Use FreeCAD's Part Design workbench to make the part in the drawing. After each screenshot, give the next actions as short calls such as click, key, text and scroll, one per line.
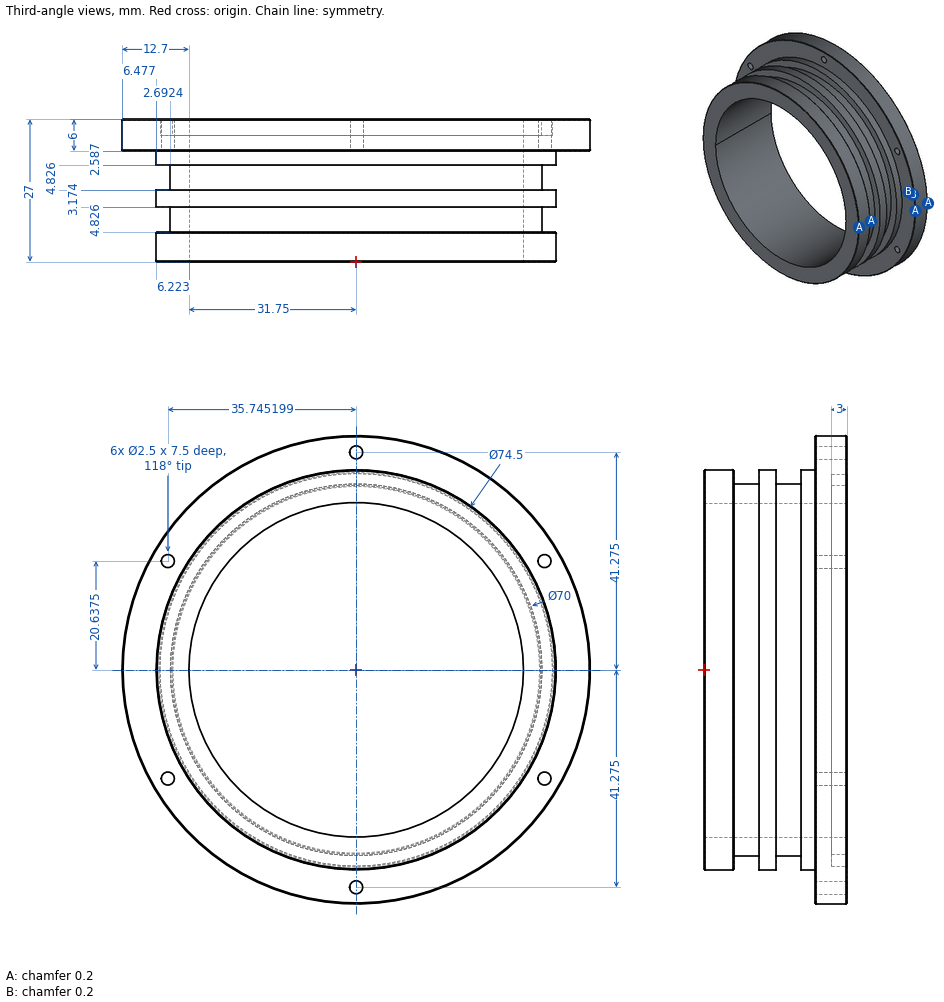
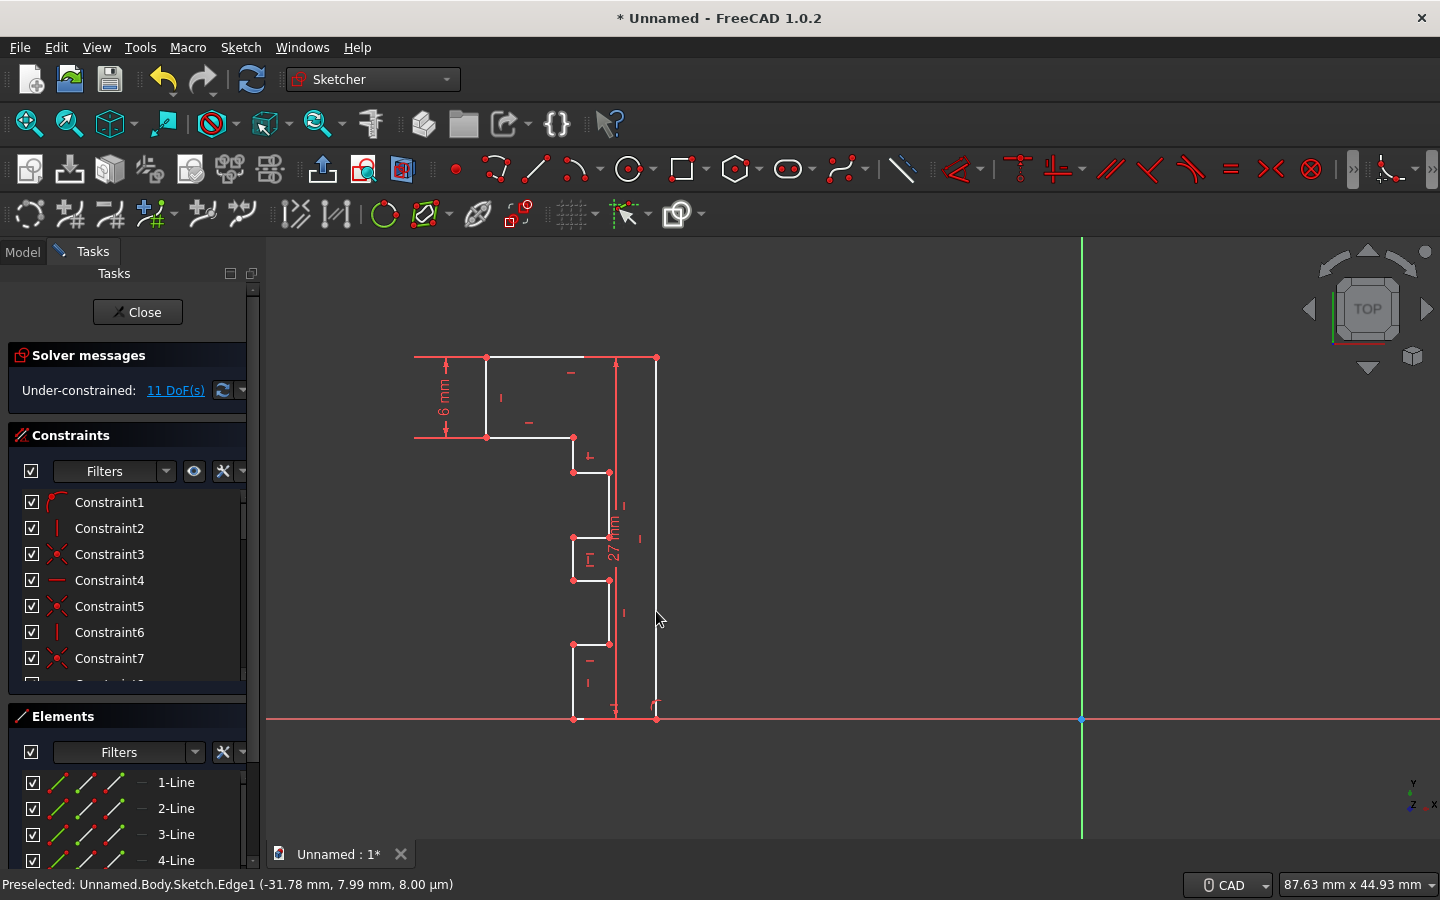
click(605, 357)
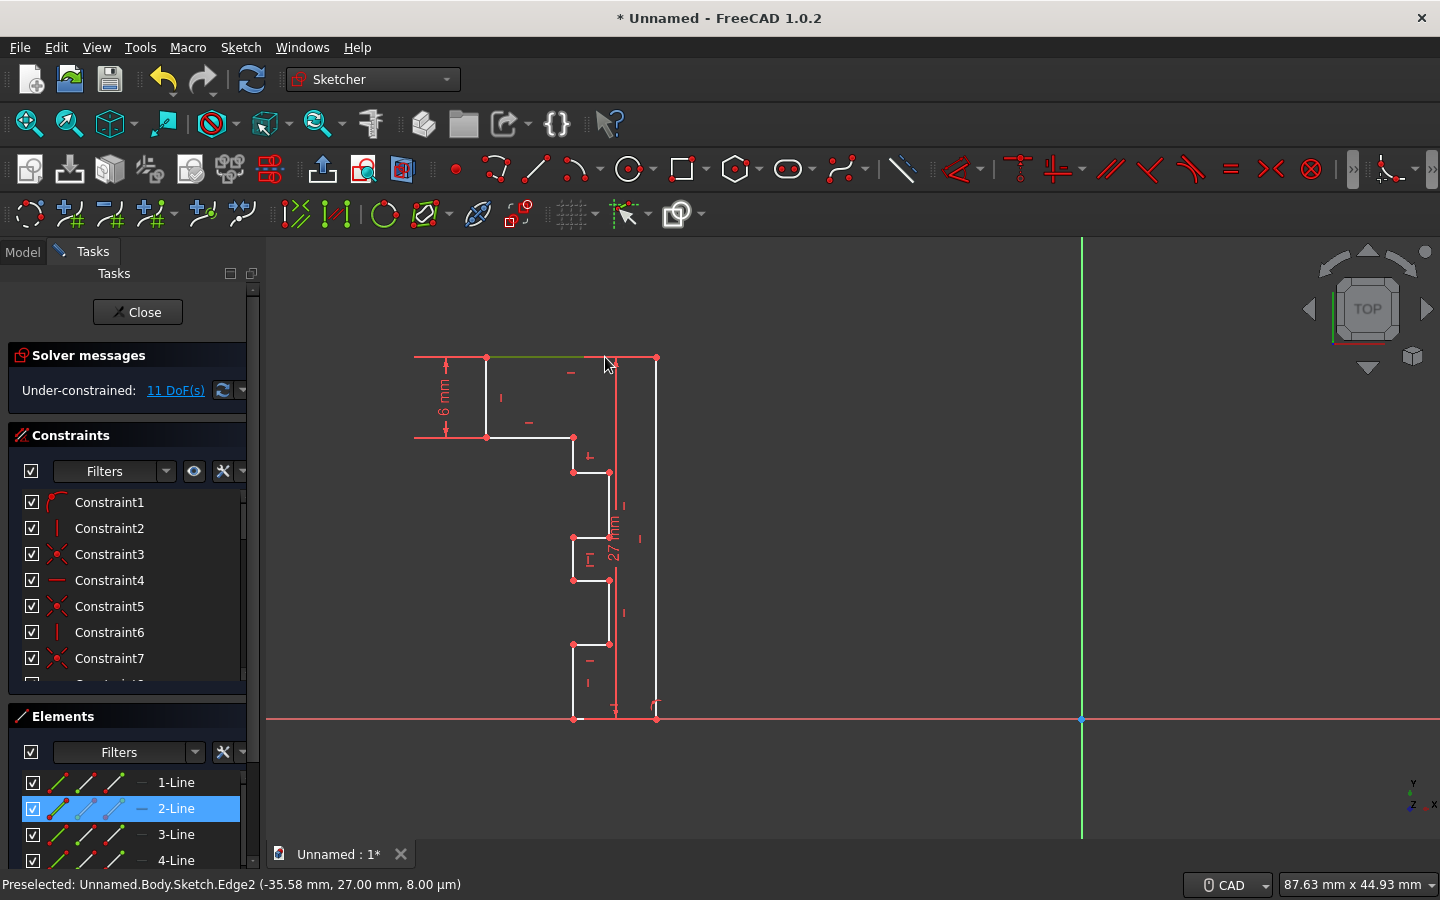
key(l)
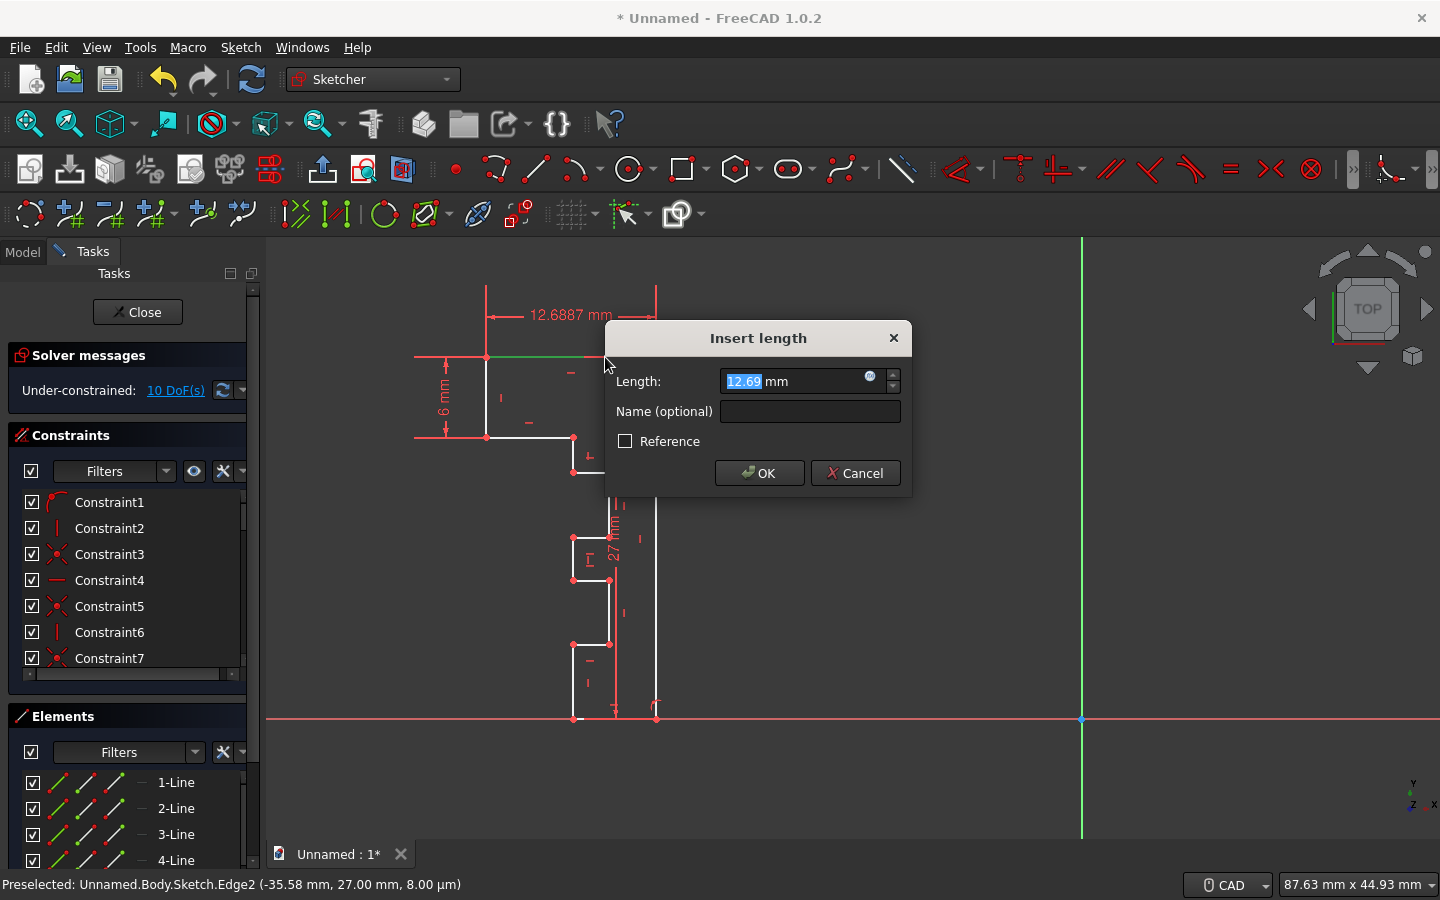
text(12.7)
key(Return)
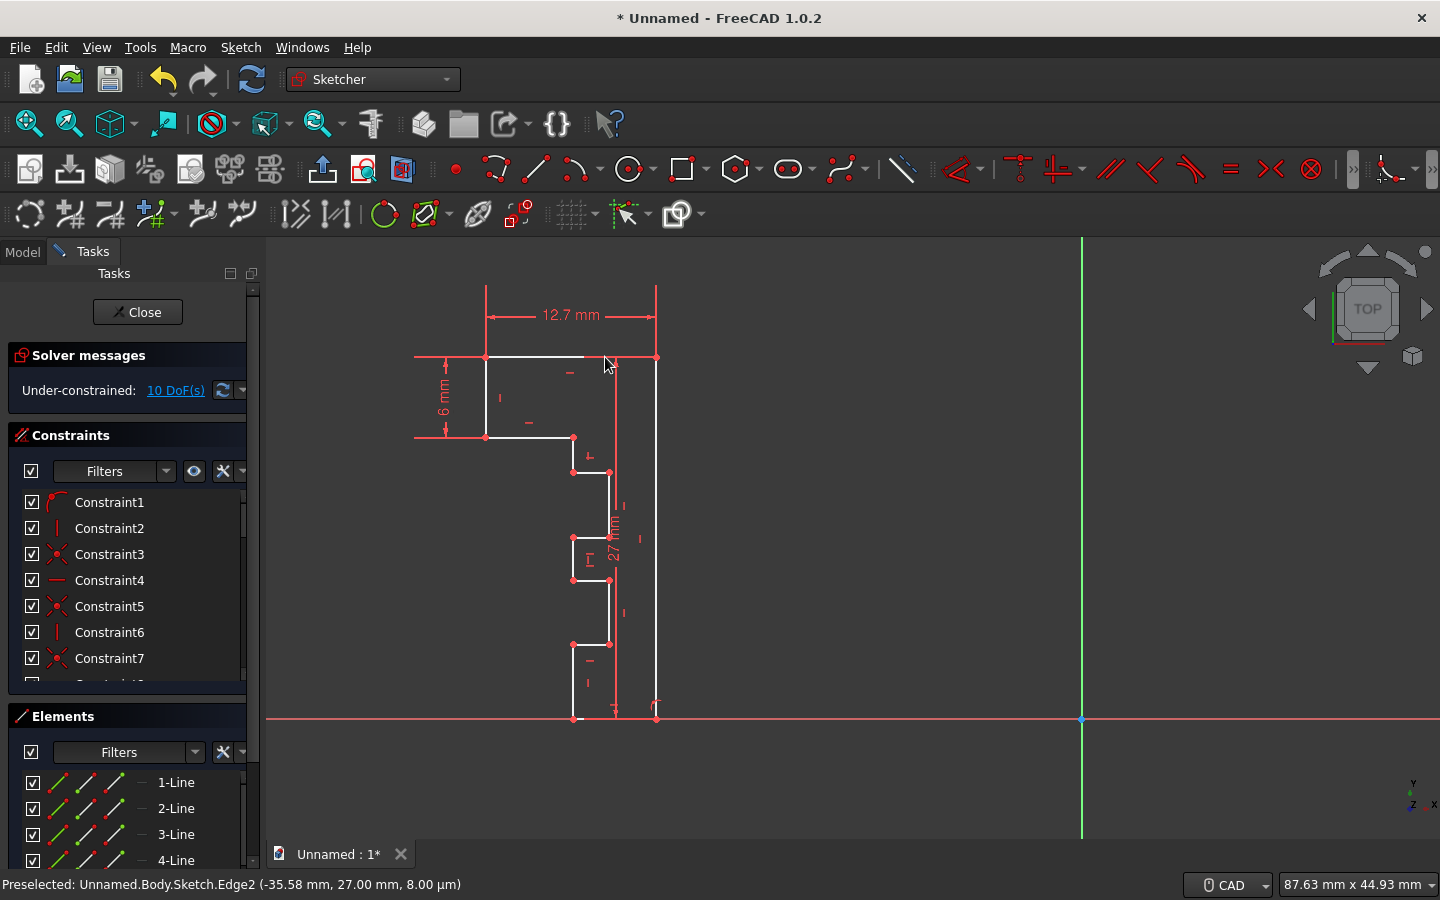
click(512, 438)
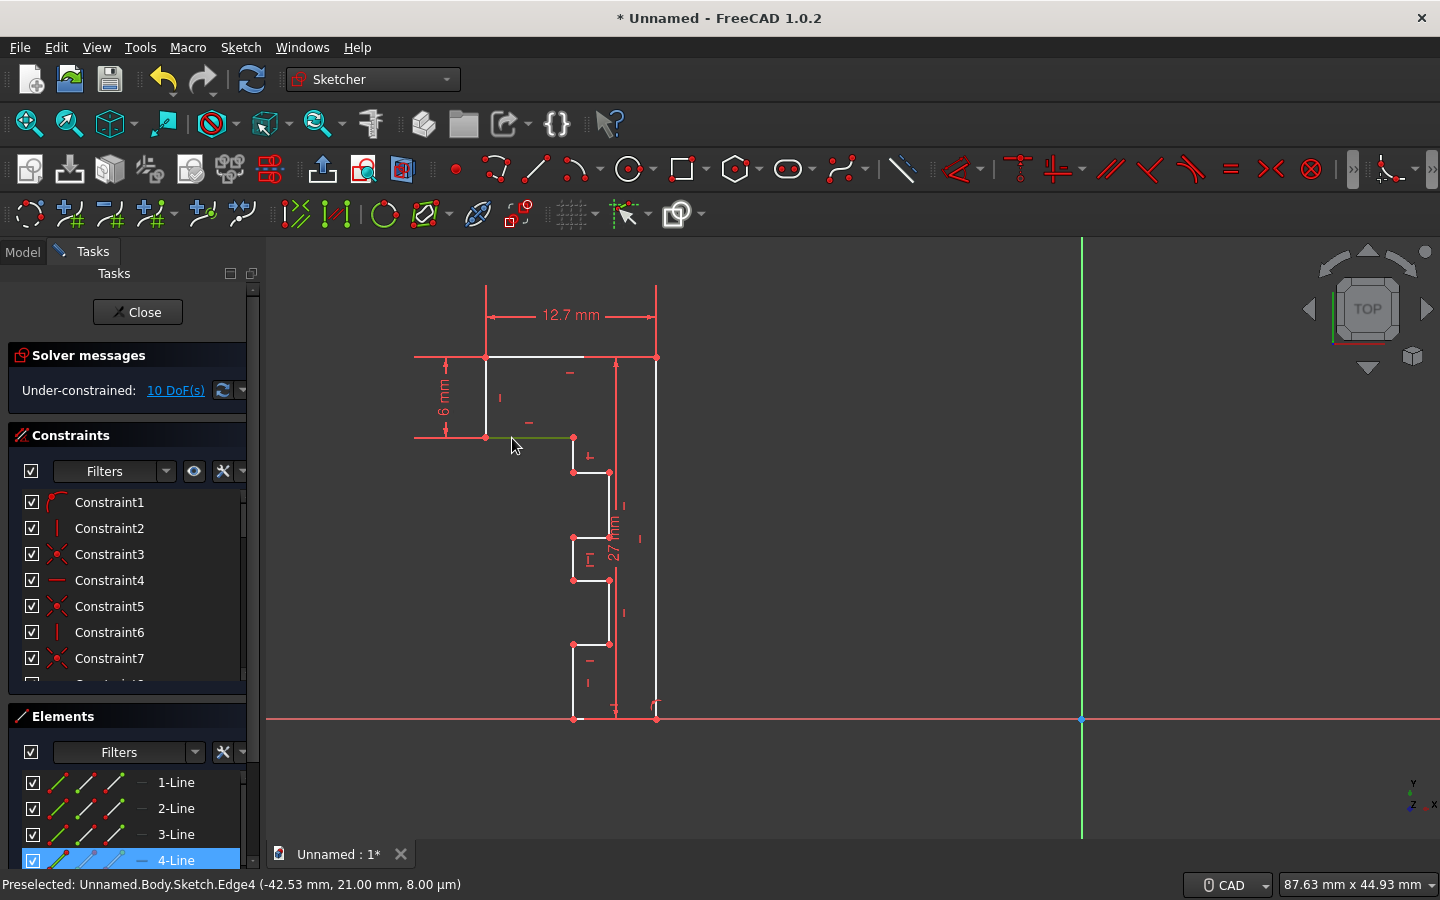
key(l)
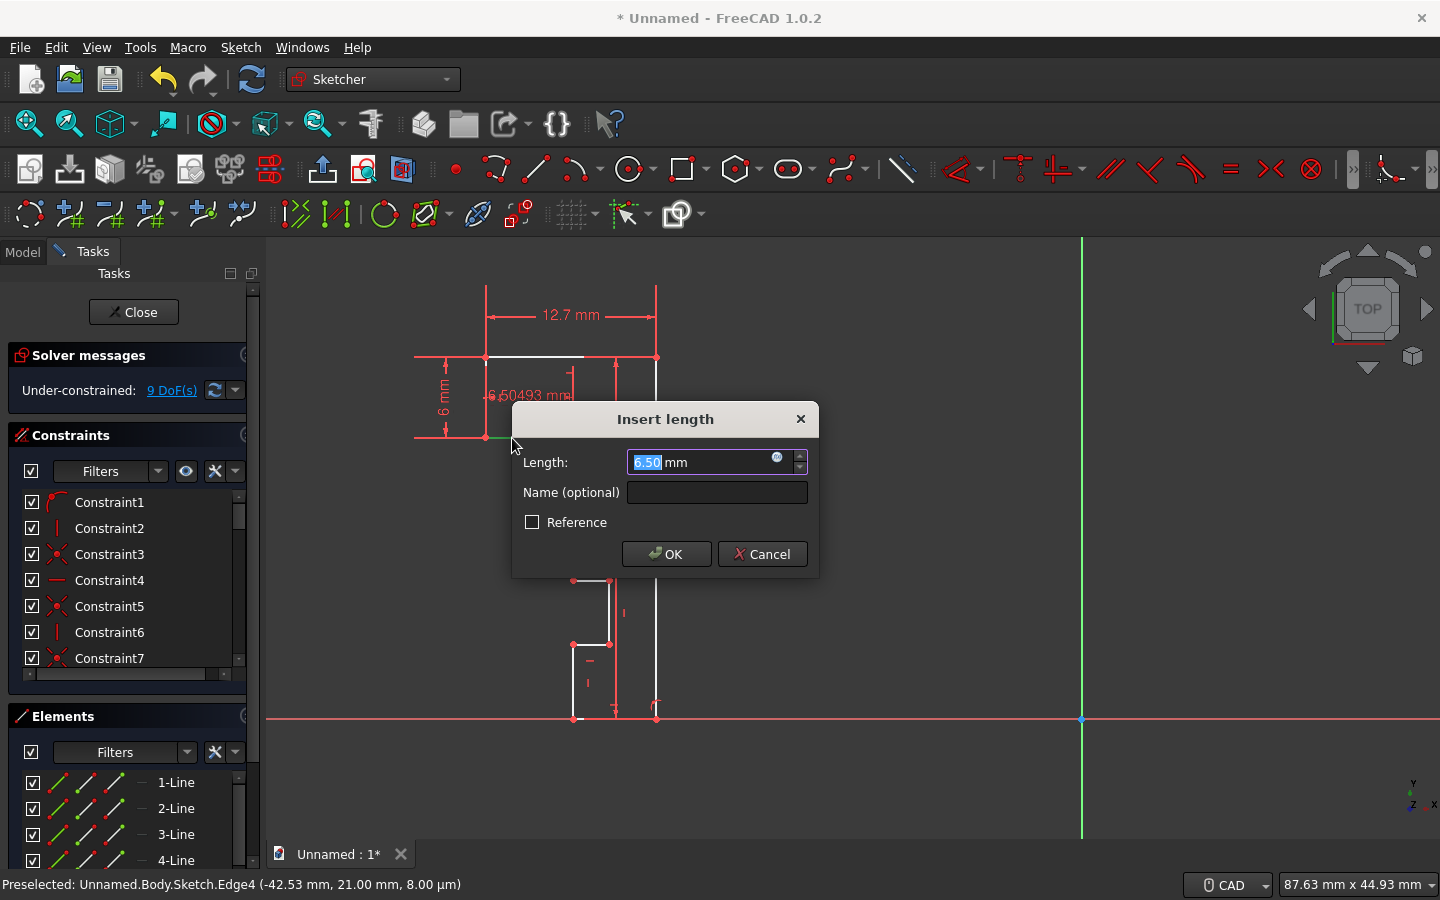
text(6.477)
key(Return)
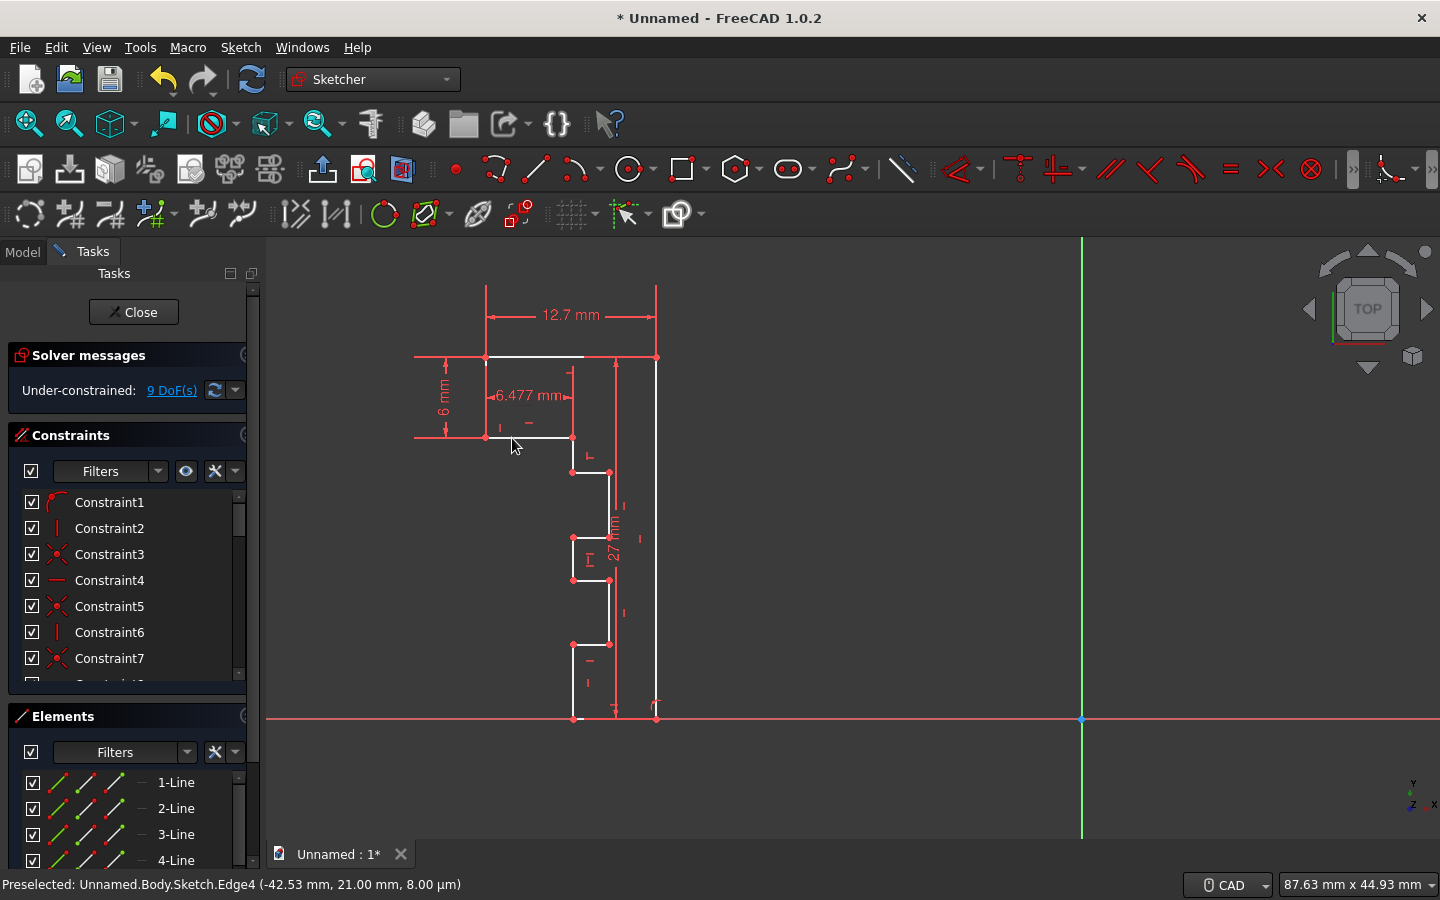
scroll(573, 448, up, 2)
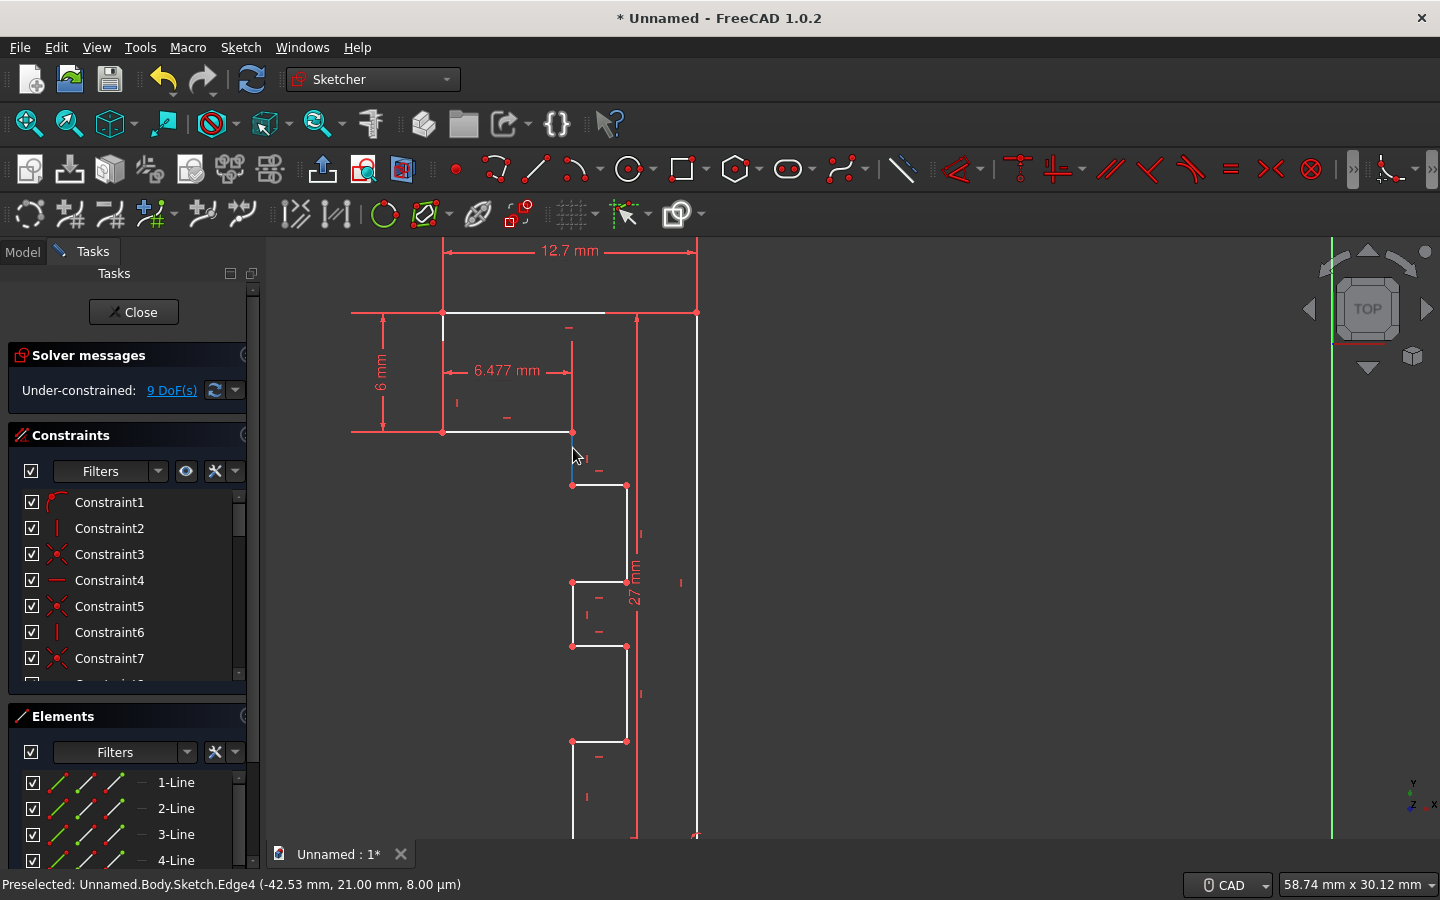
click(572, 448)